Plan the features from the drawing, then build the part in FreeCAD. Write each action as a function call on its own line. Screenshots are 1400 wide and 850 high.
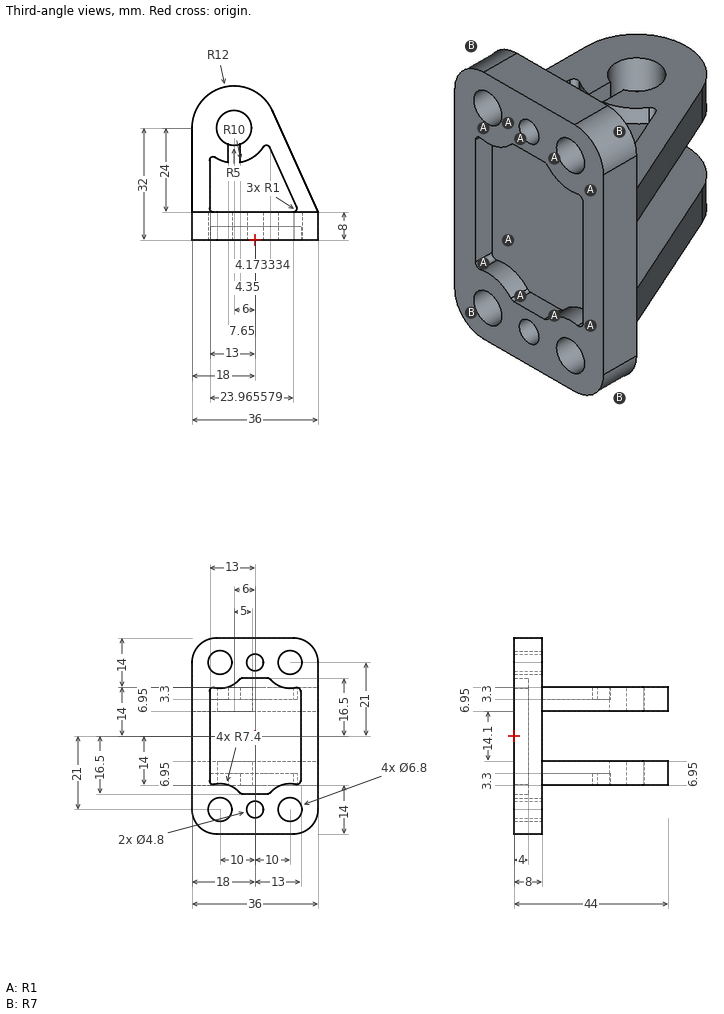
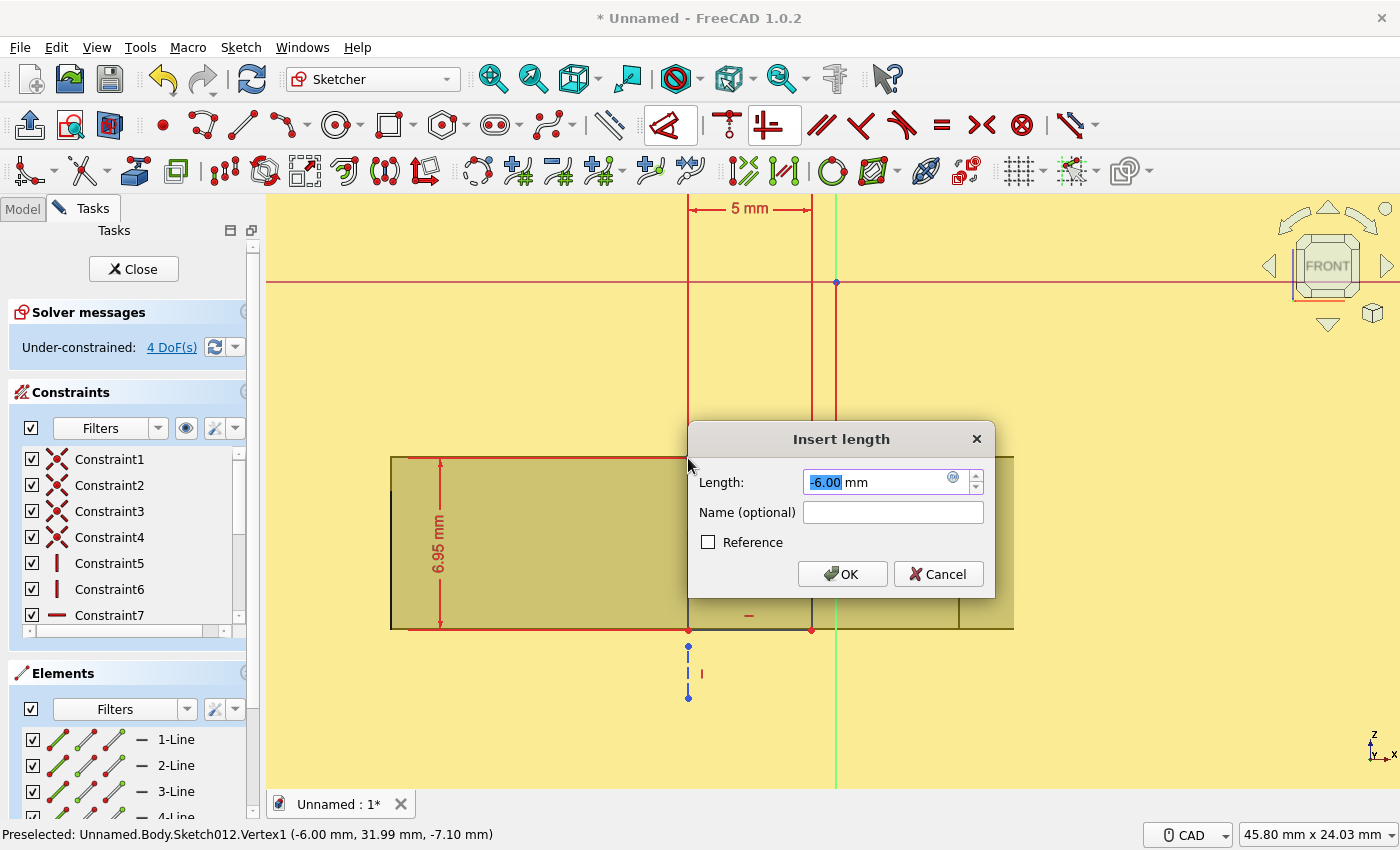
text(-6)
key(Return)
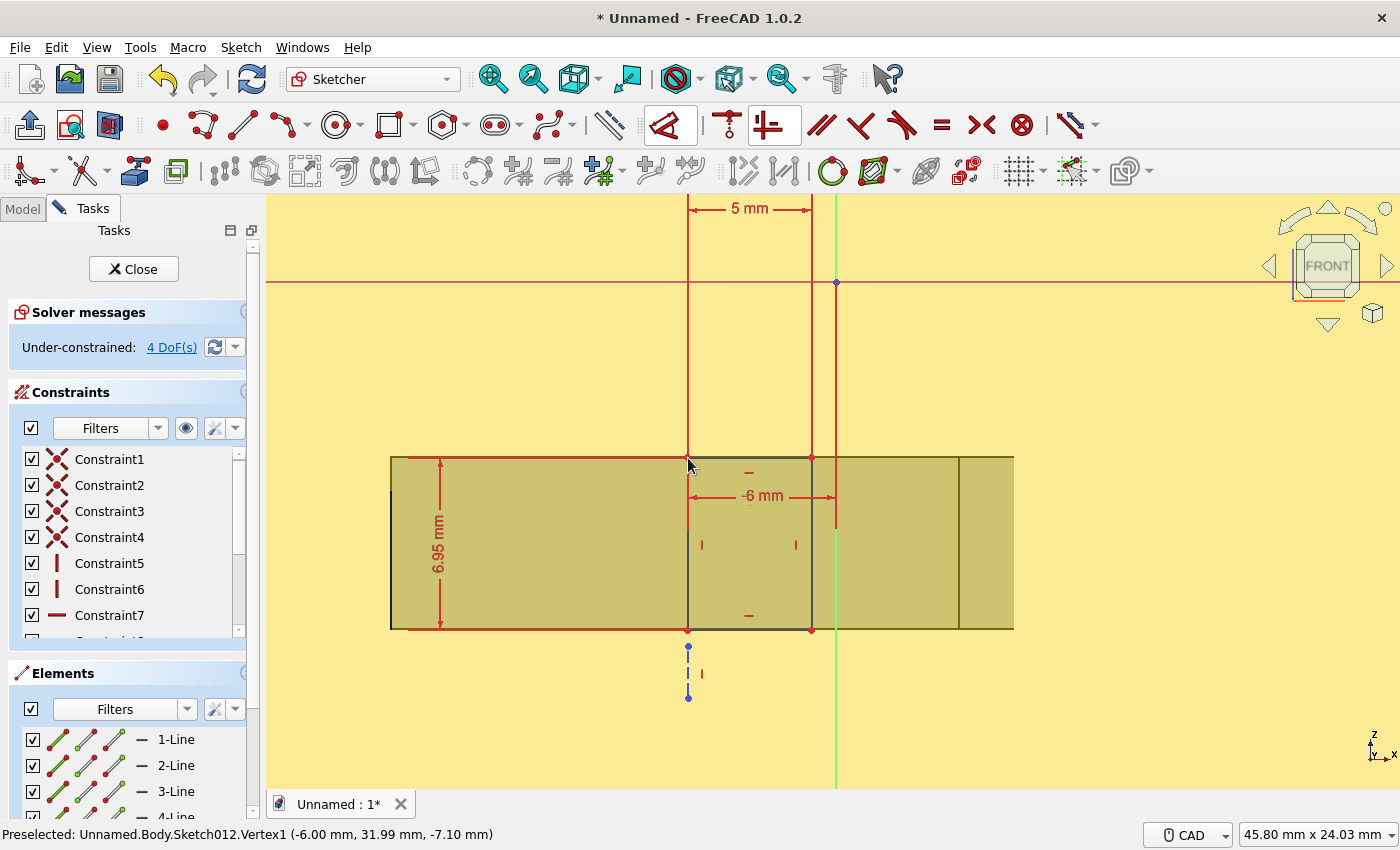
click(688, 647)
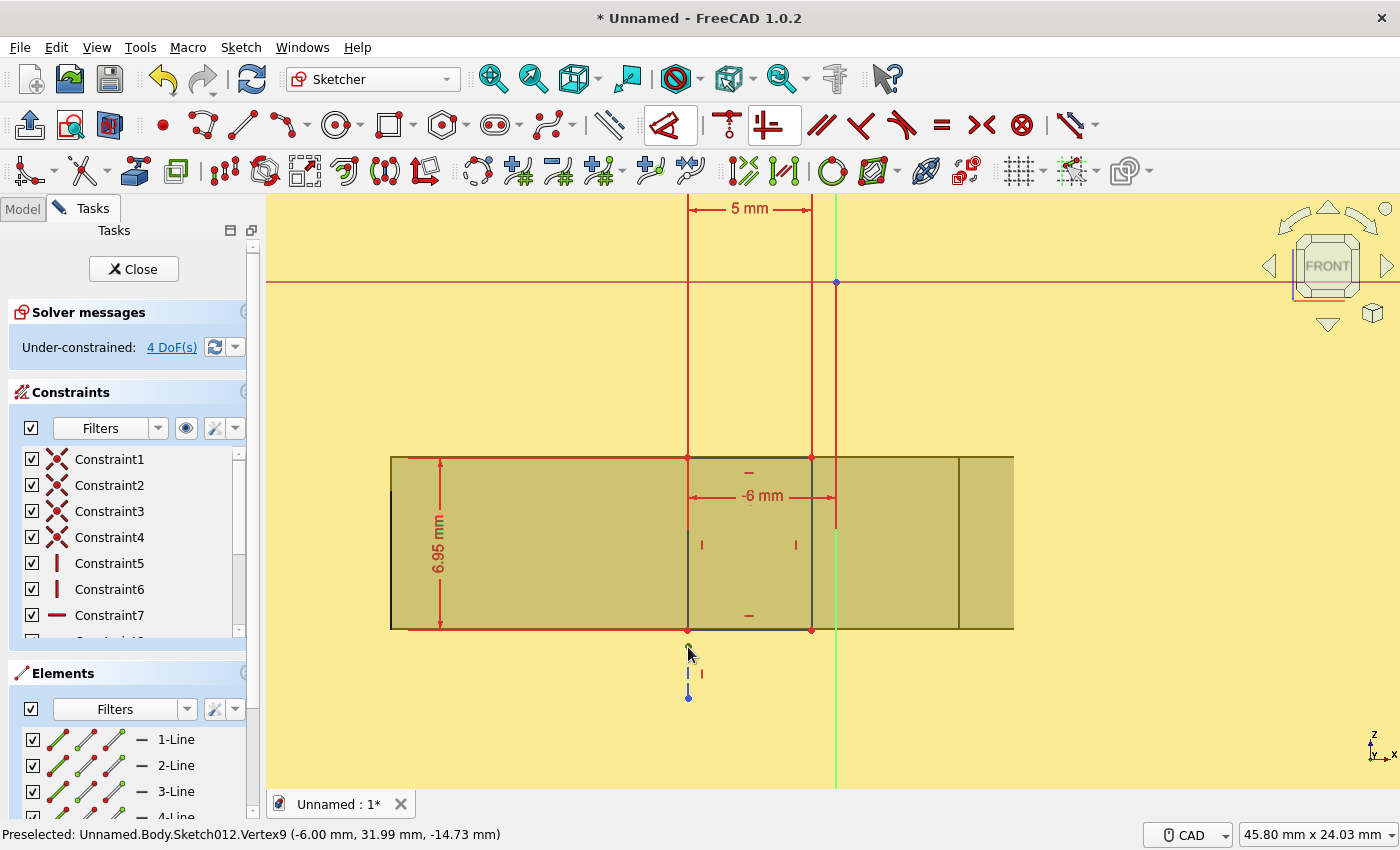
key(l)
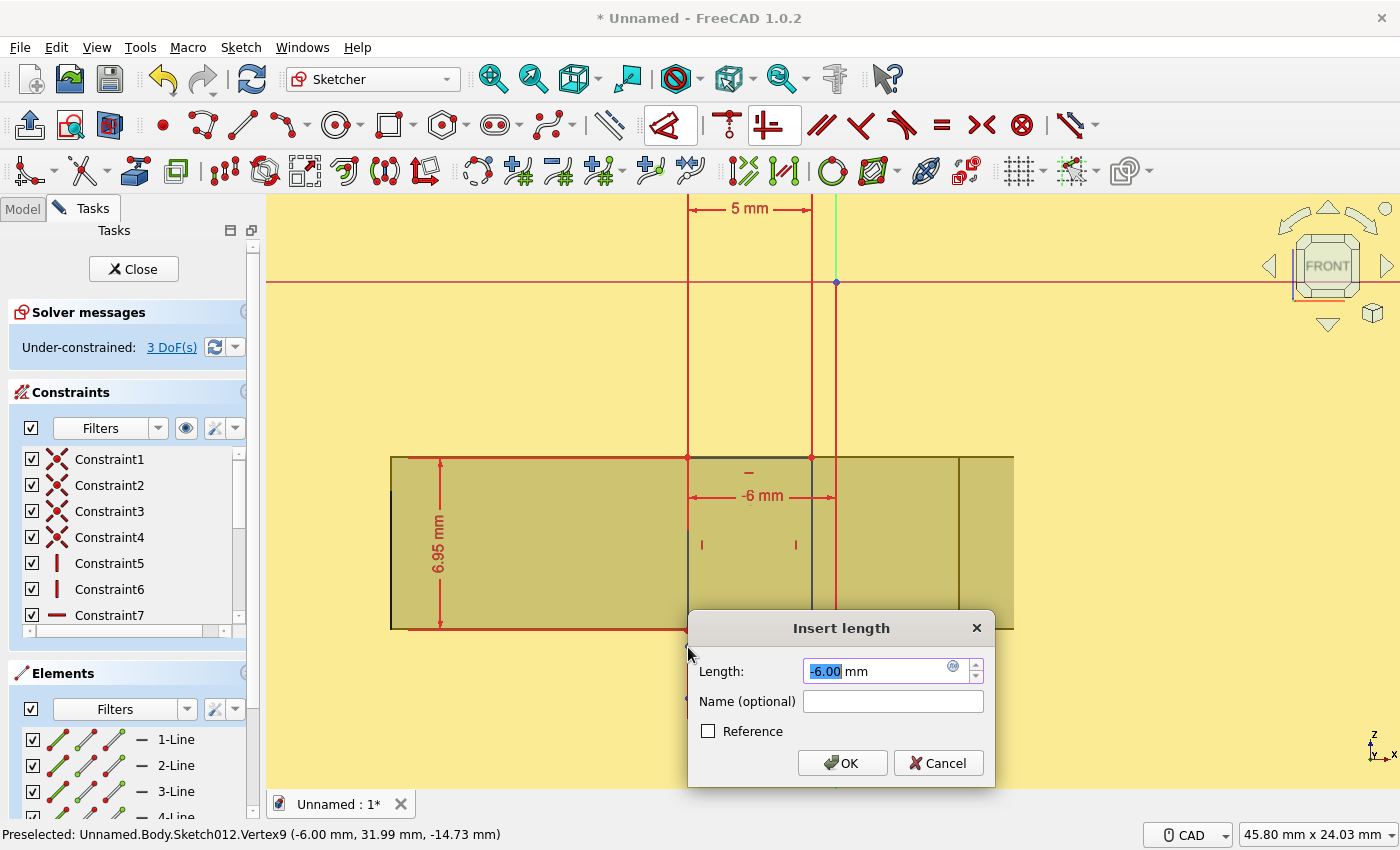
text(-6)
key(Return)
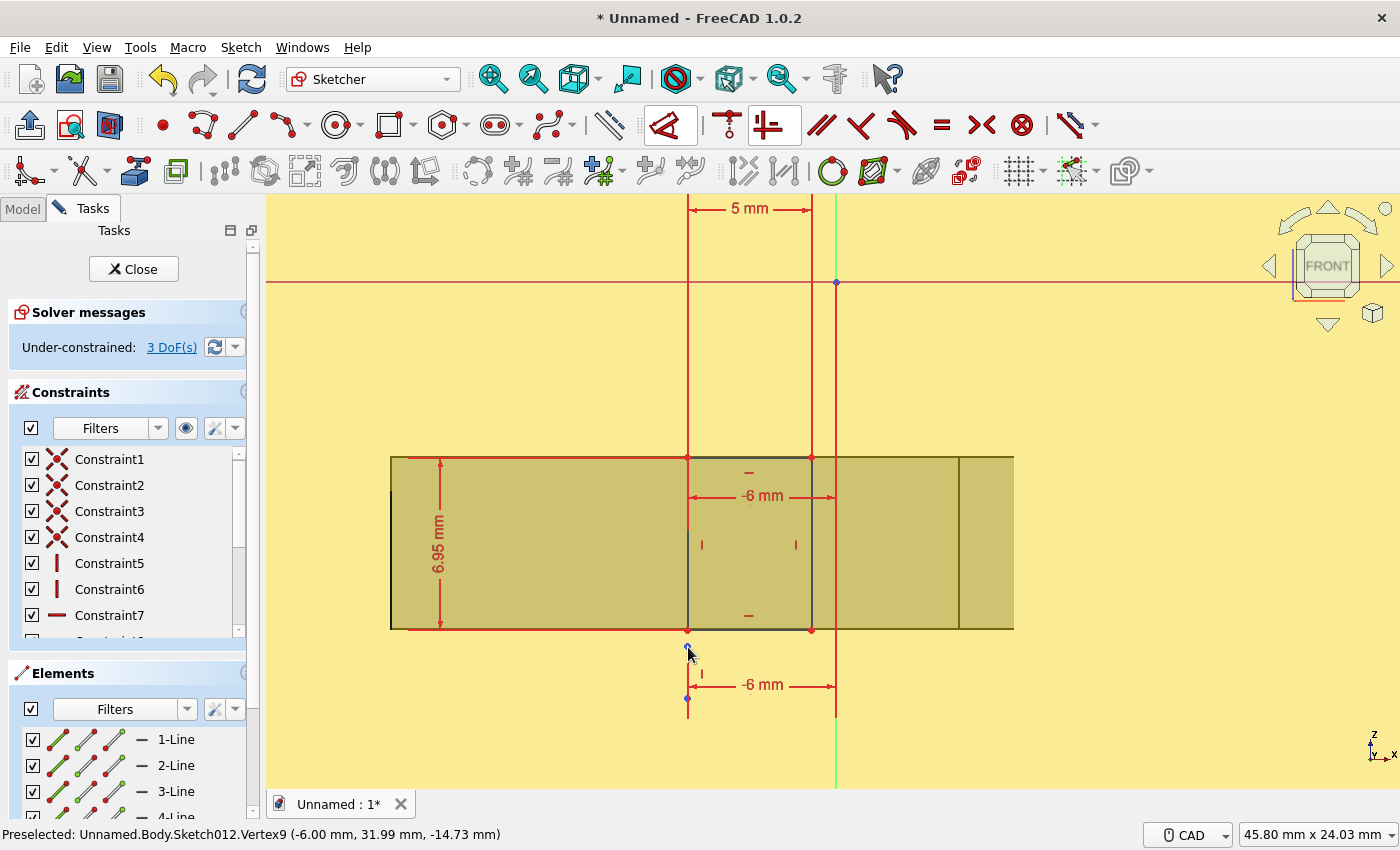
click(688, 630)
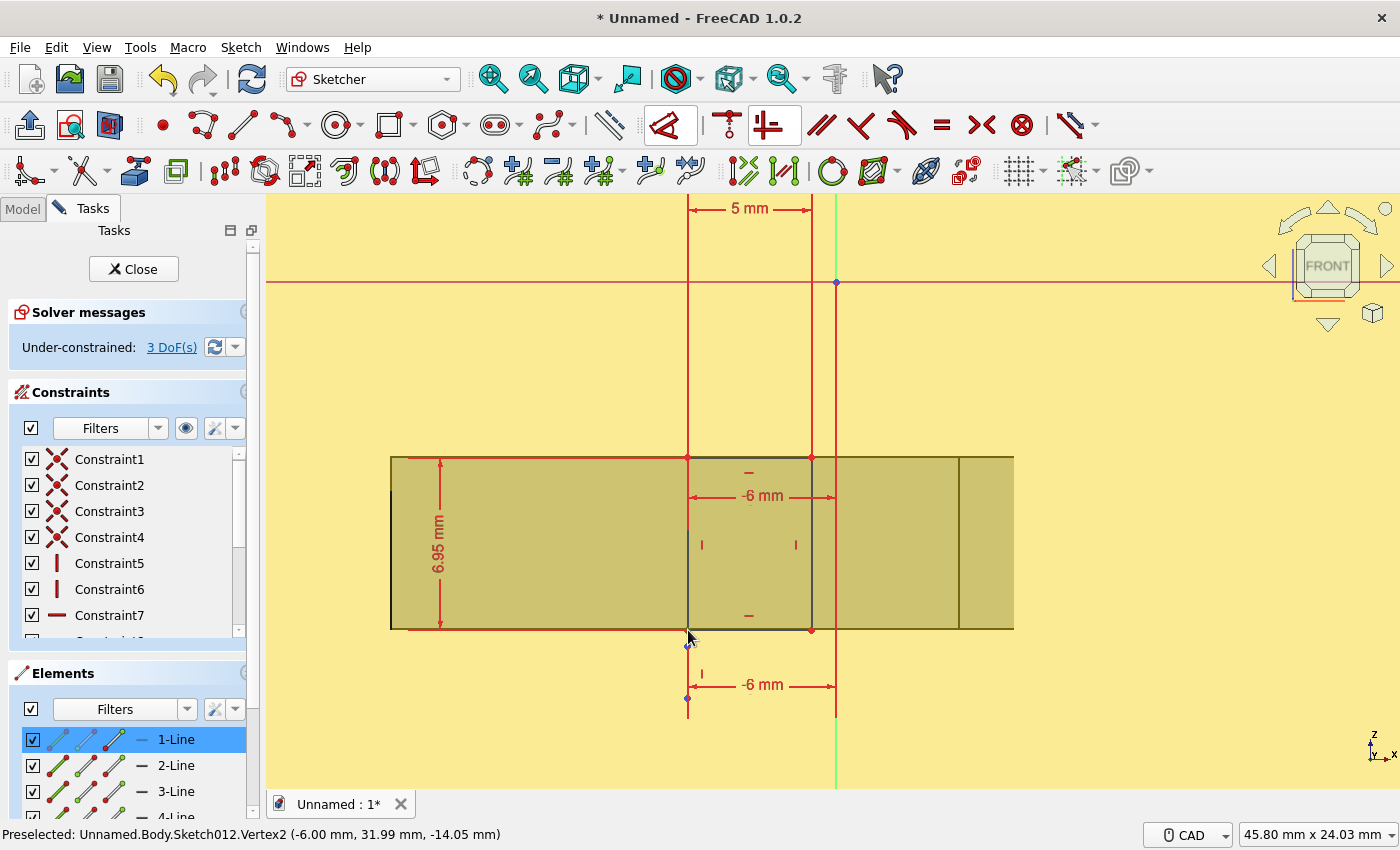
key(i)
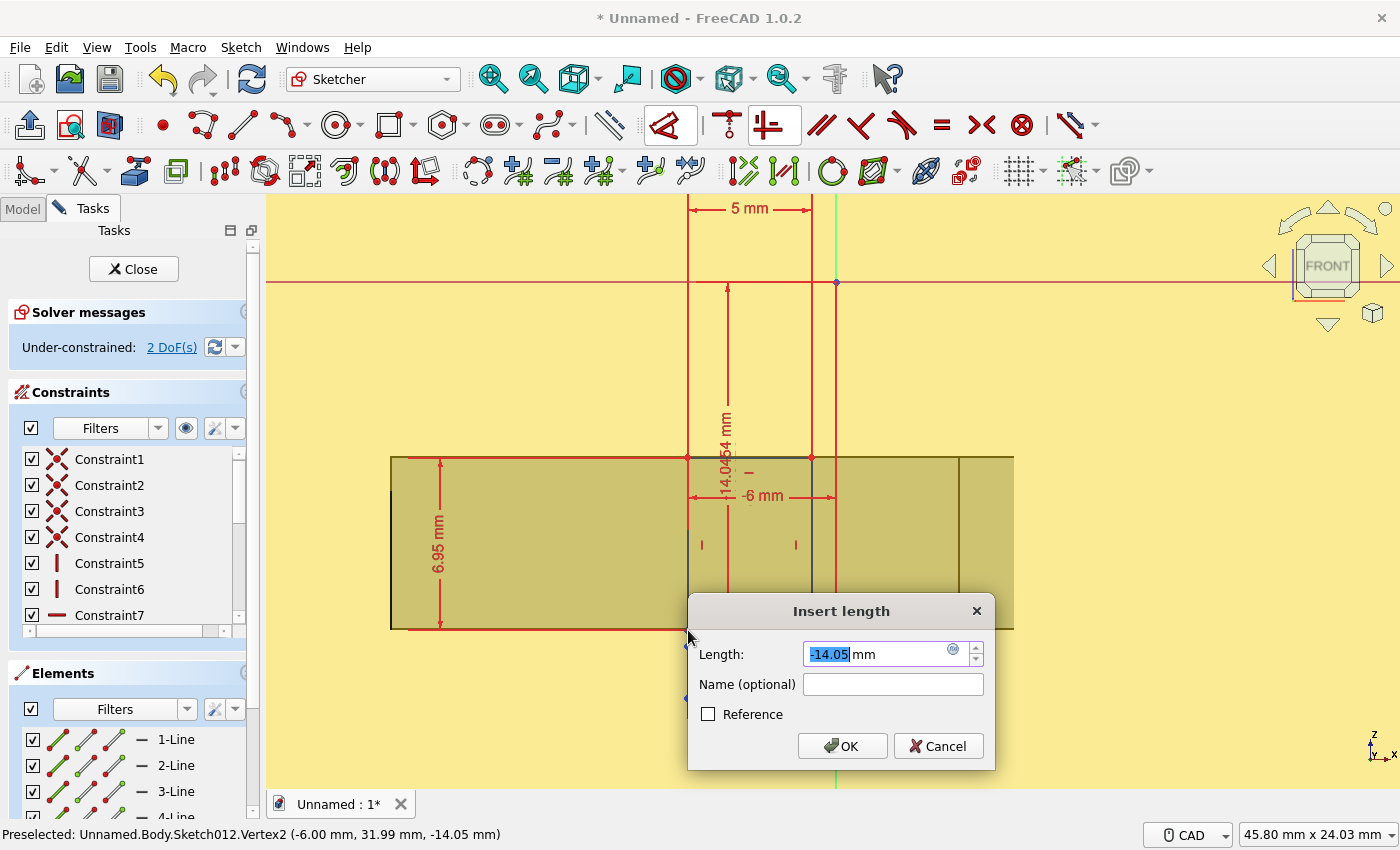
text(-14)
key(Return)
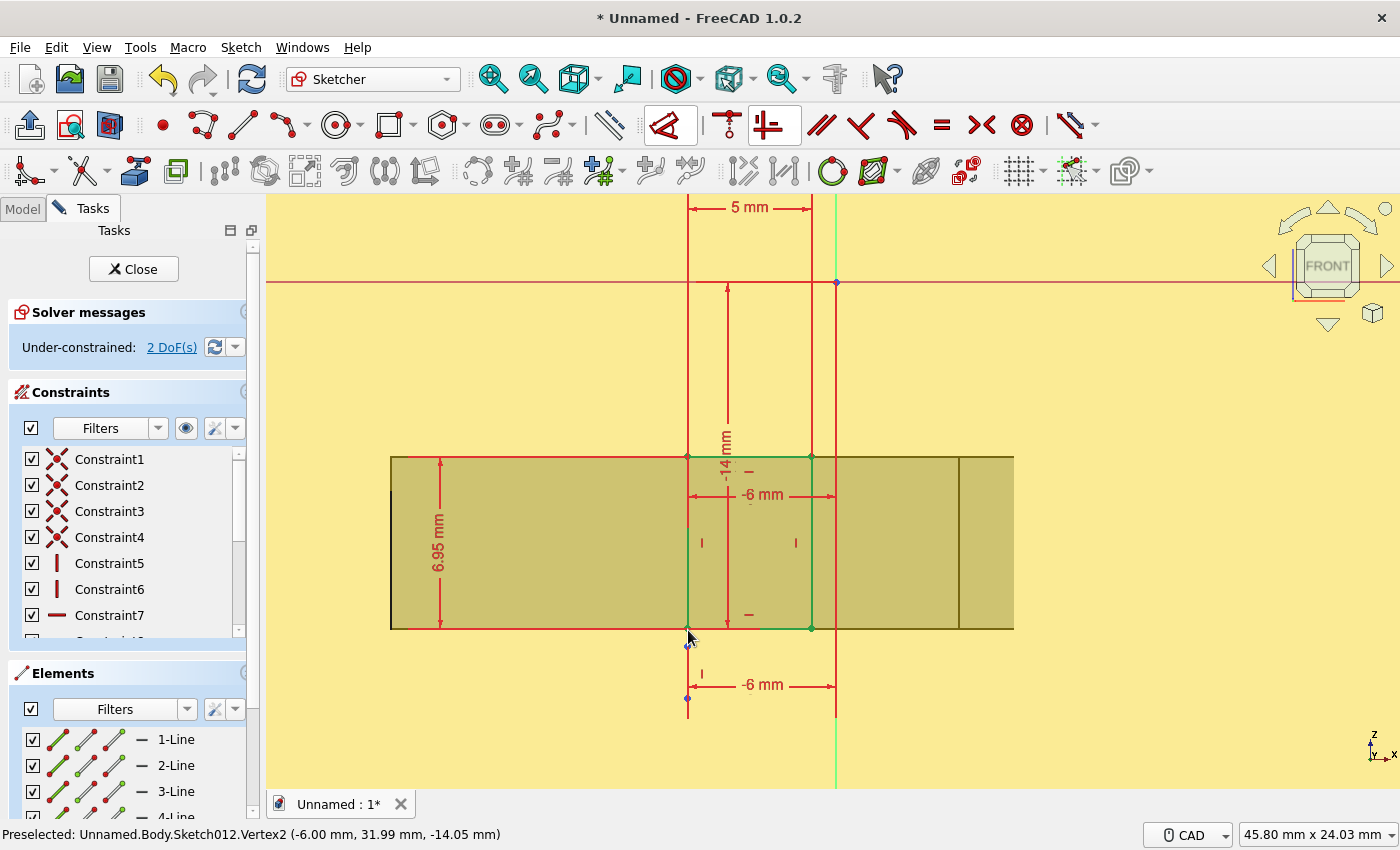
click(134, 269)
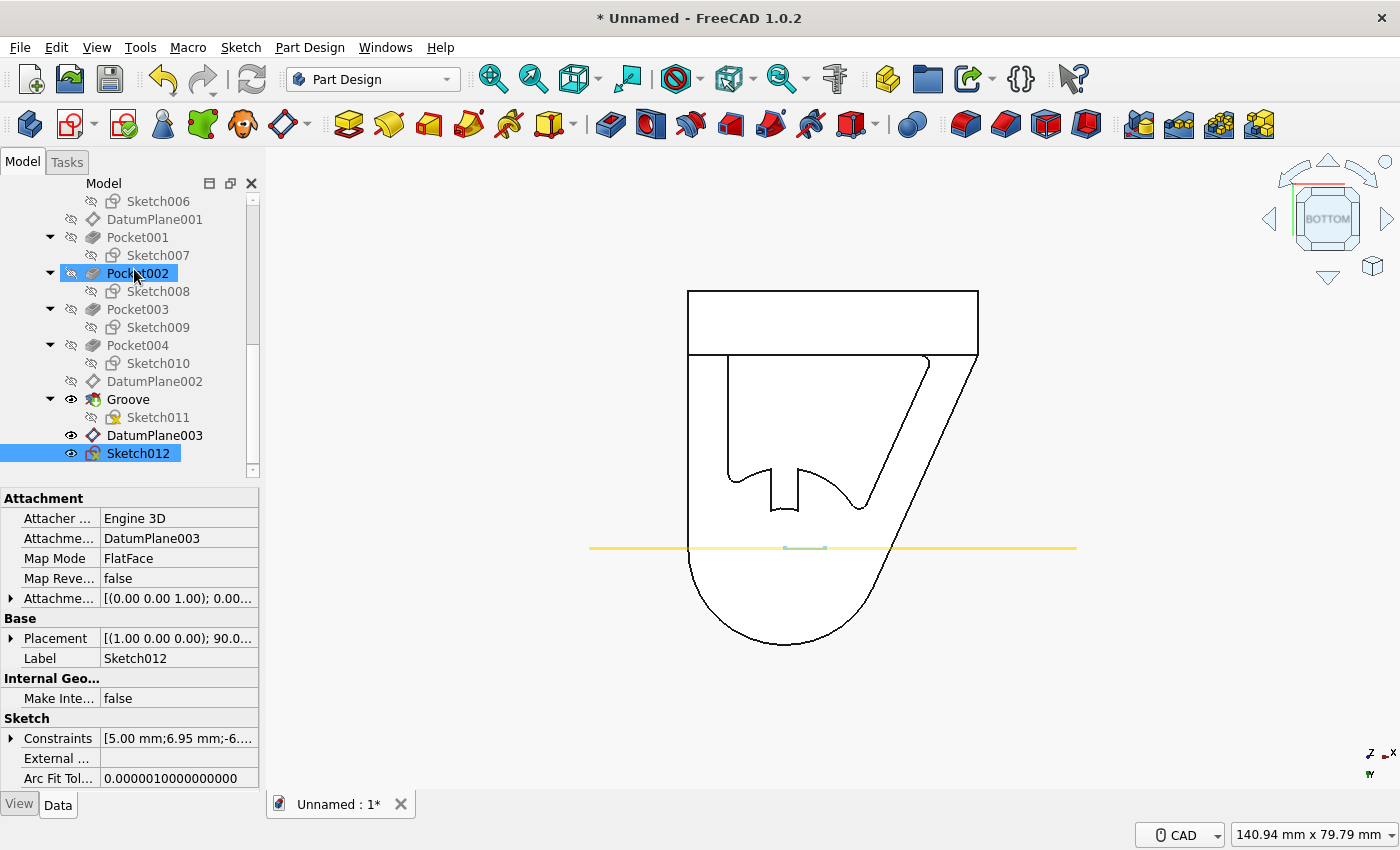
click(692, 124)